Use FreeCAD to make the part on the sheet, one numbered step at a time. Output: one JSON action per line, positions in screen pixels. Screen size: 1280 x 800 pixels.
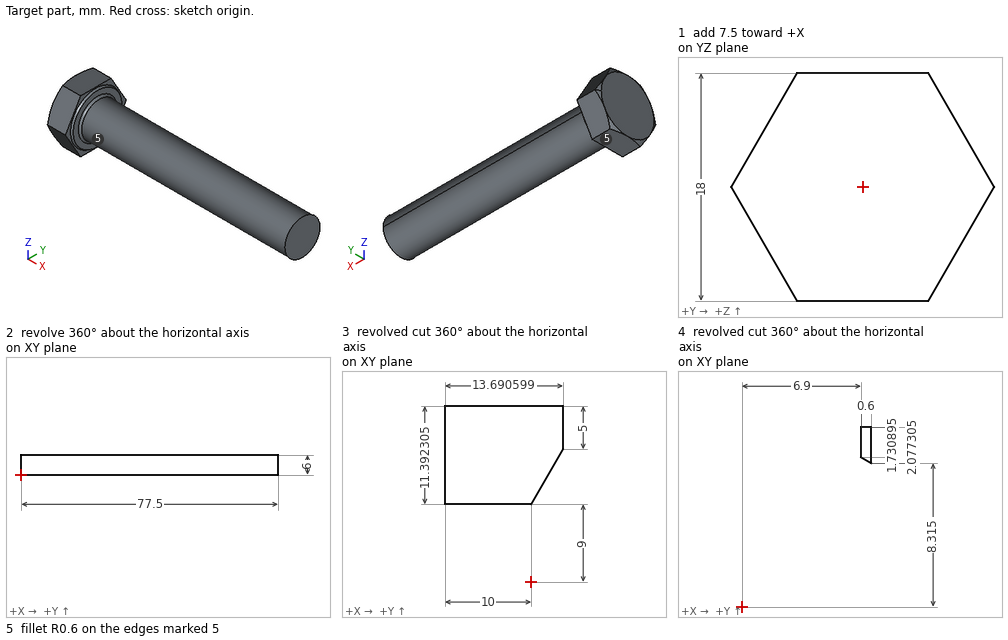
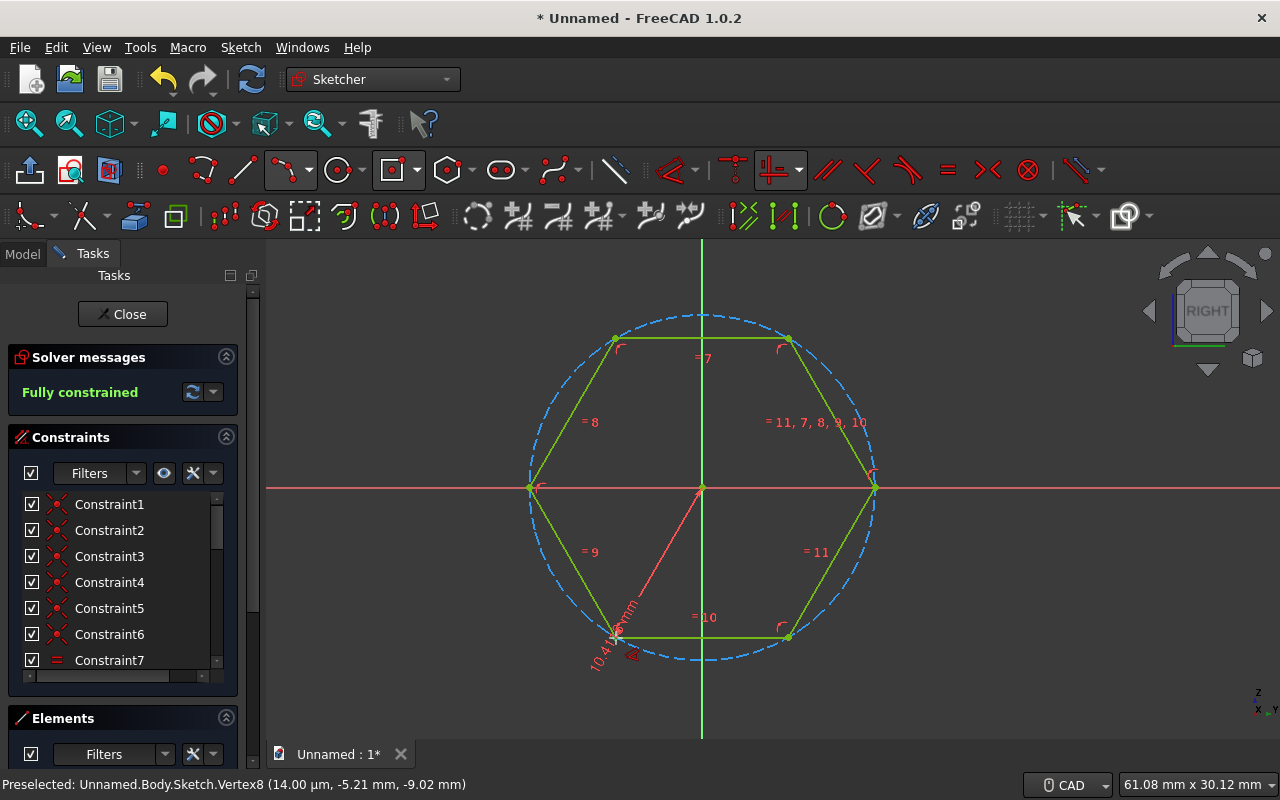
{"action": "left_click", "coordinate": [789, 338]}
{"action": "left_click", "coordinate": [871, 383]}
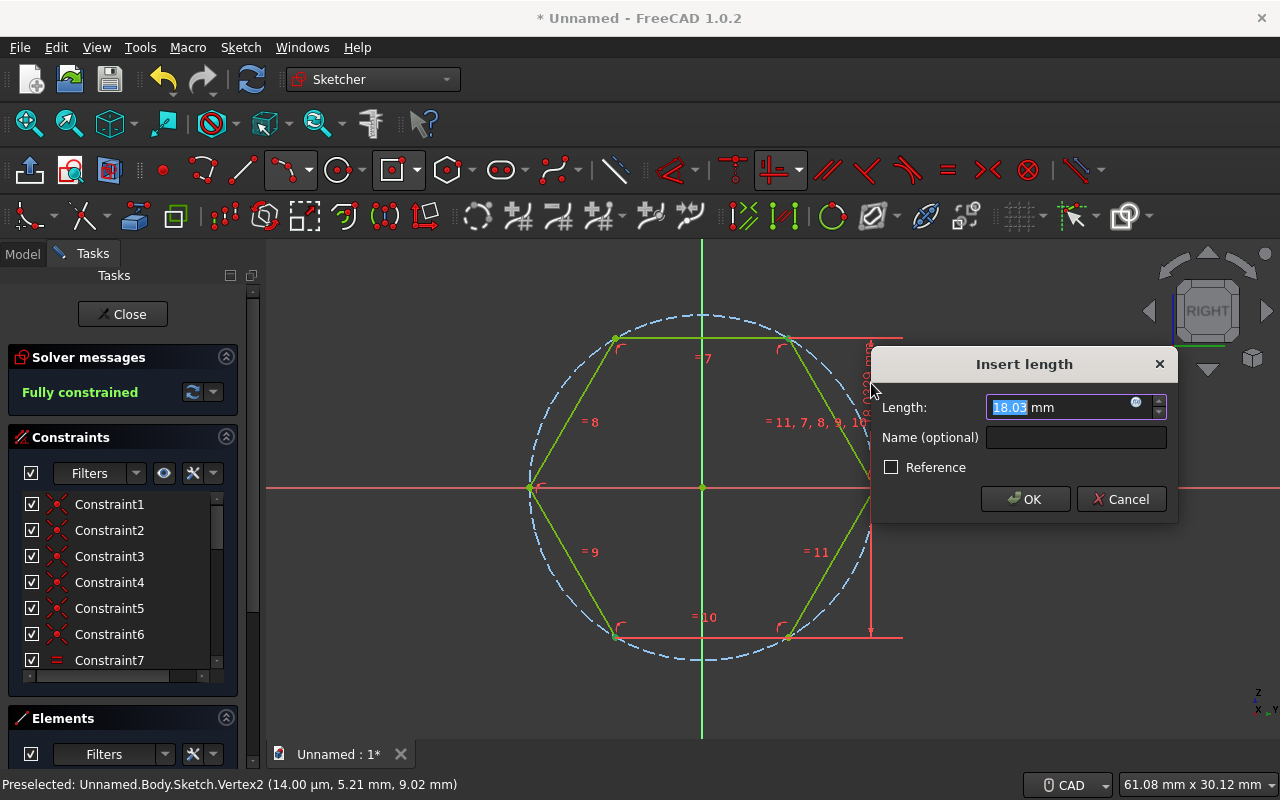
{"action": "type", "text": "18"}
{"action": "key", "text": "Return"}
{"action": "key", "text": "Escape"}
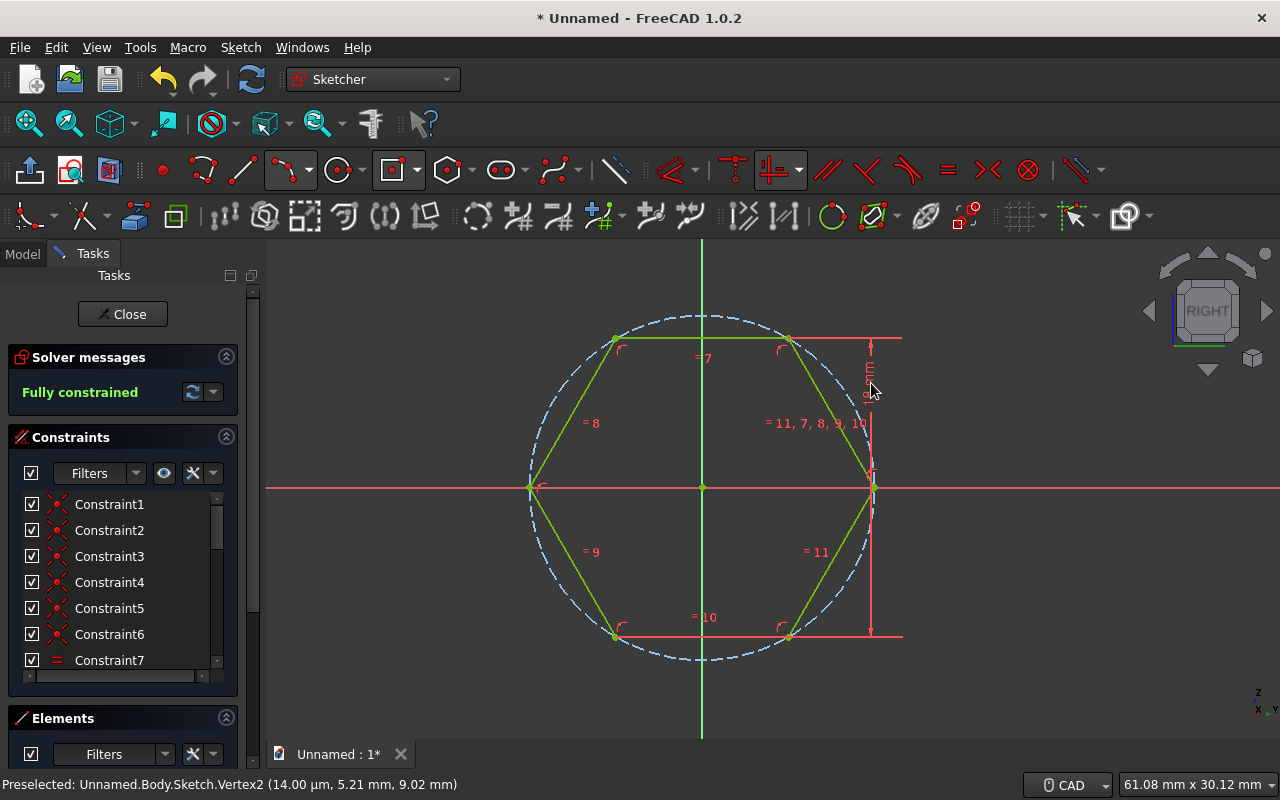
{"action": "left_click", "coordinate": [123, 314]}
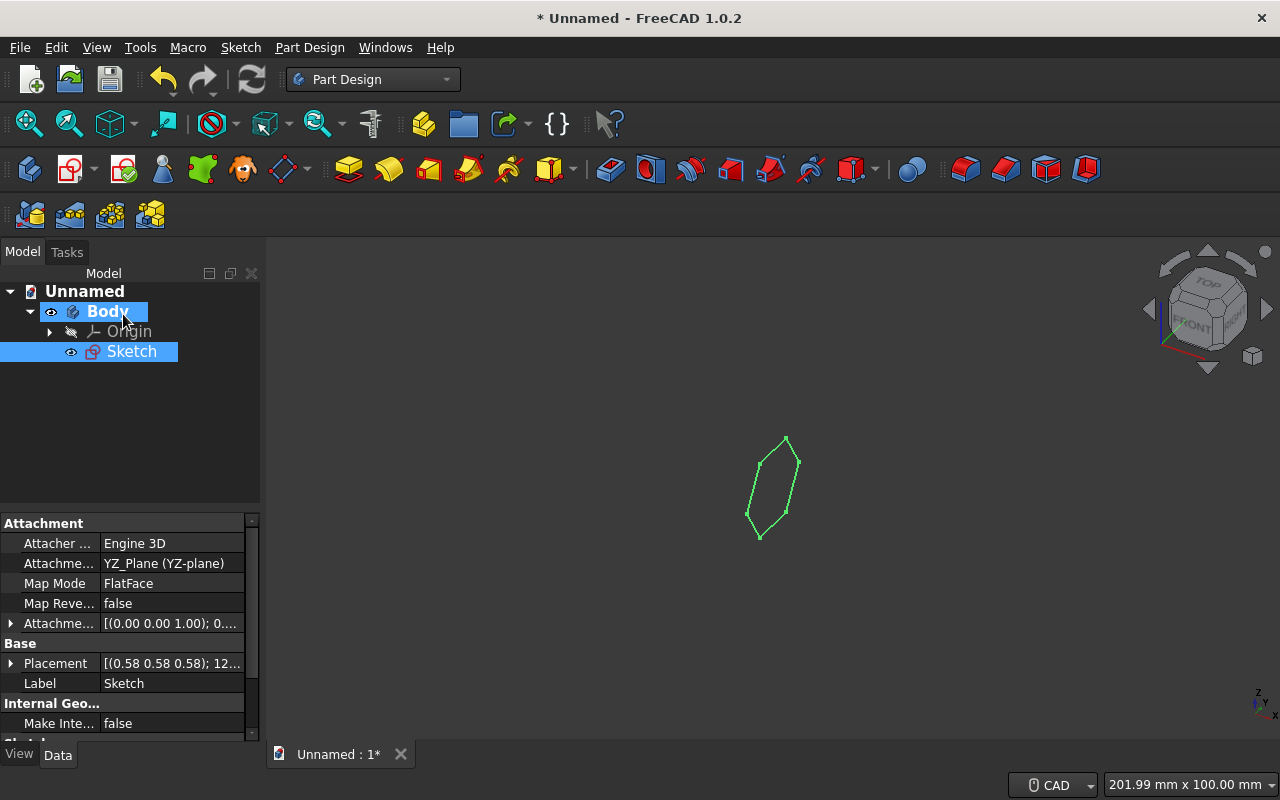
{"action": "left_click", "coordinate": [350, 170]}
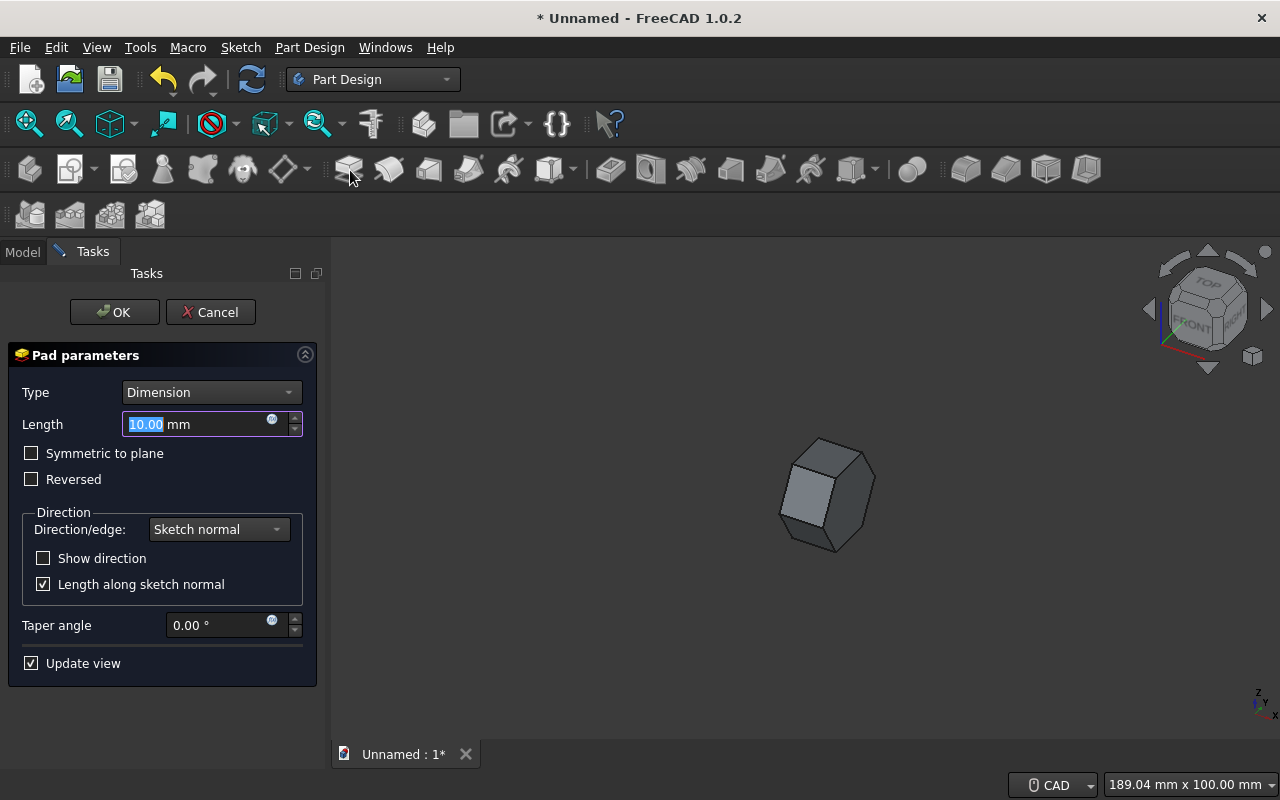
{"action": "type", "text": "7.5"}
{"action": "key", "text": "Tab"}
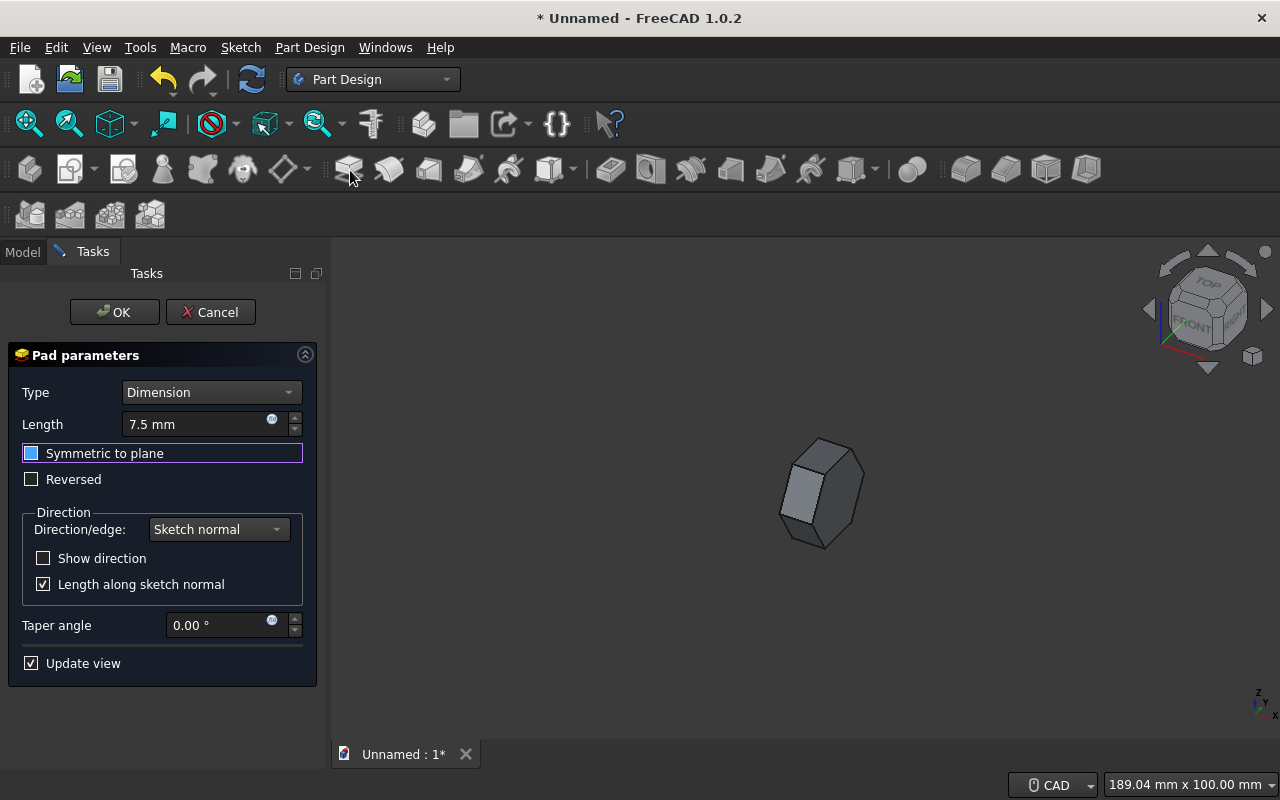
{"action": "left_click", "coordinate": [115, 312]}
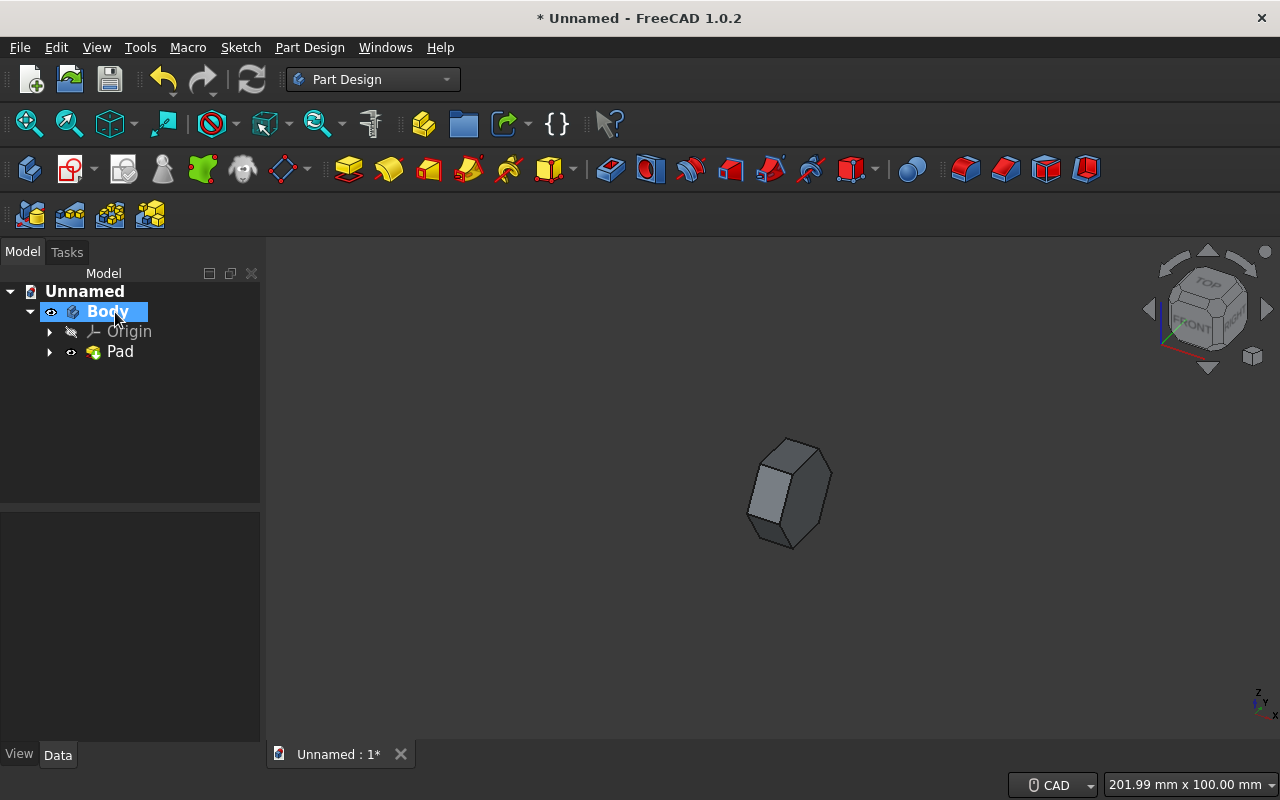
{"action": "left_click", "coordinate": [30, 124]}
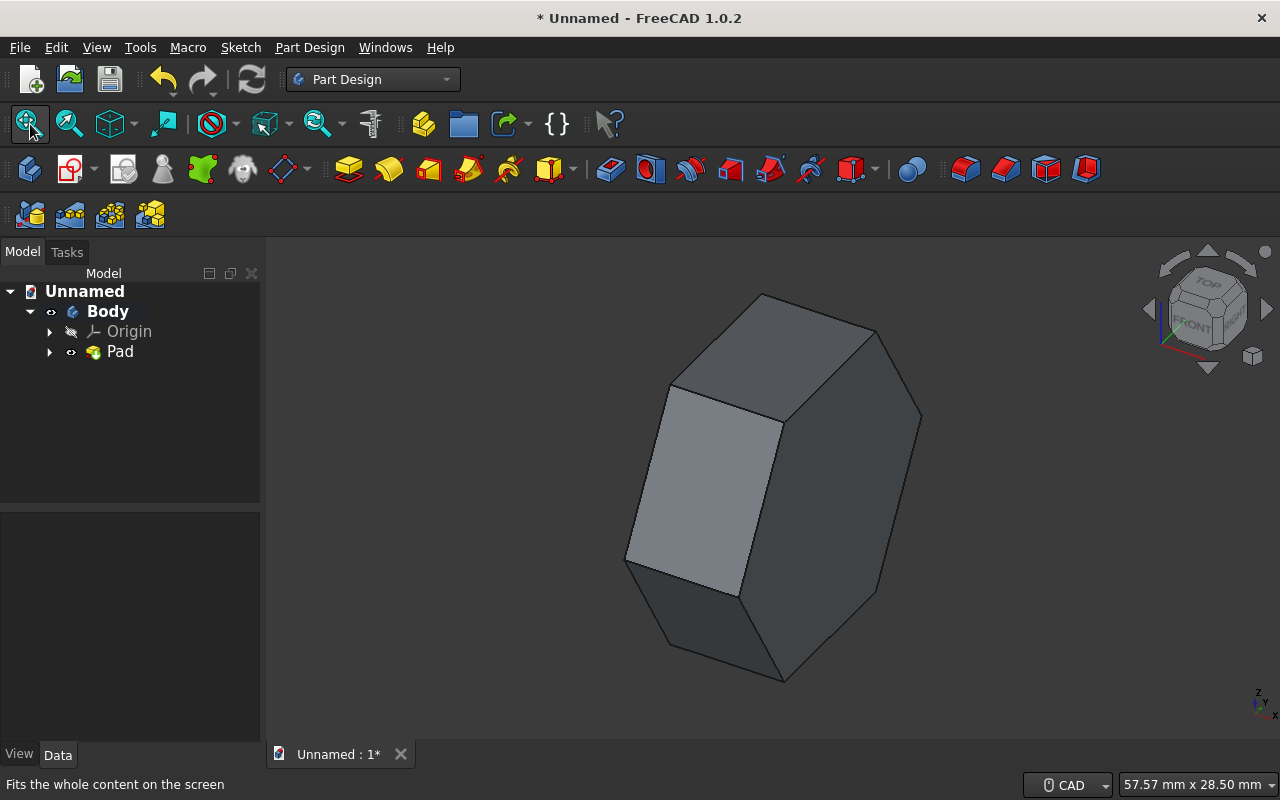
{"action": "left_click", "coordinate": [70, 170]}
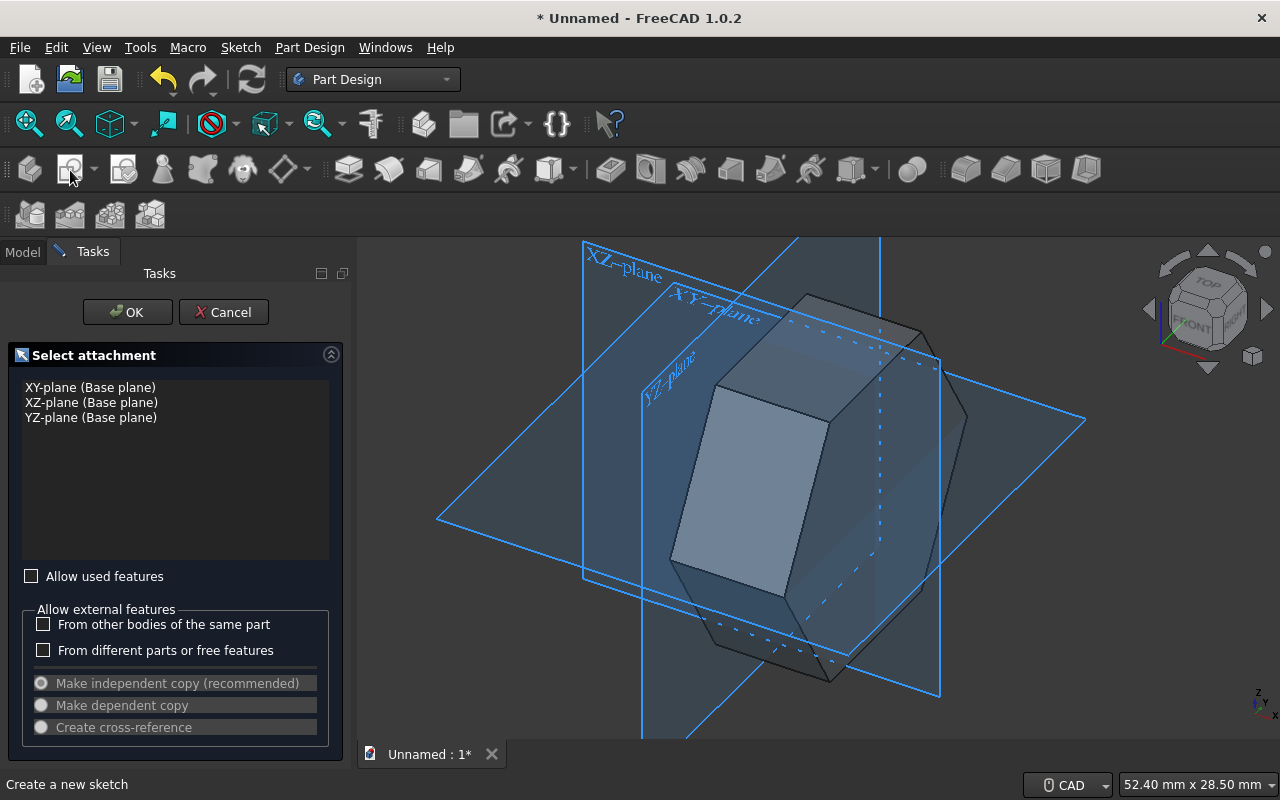
{"action": "left_click", "coordinate": [82, 388]}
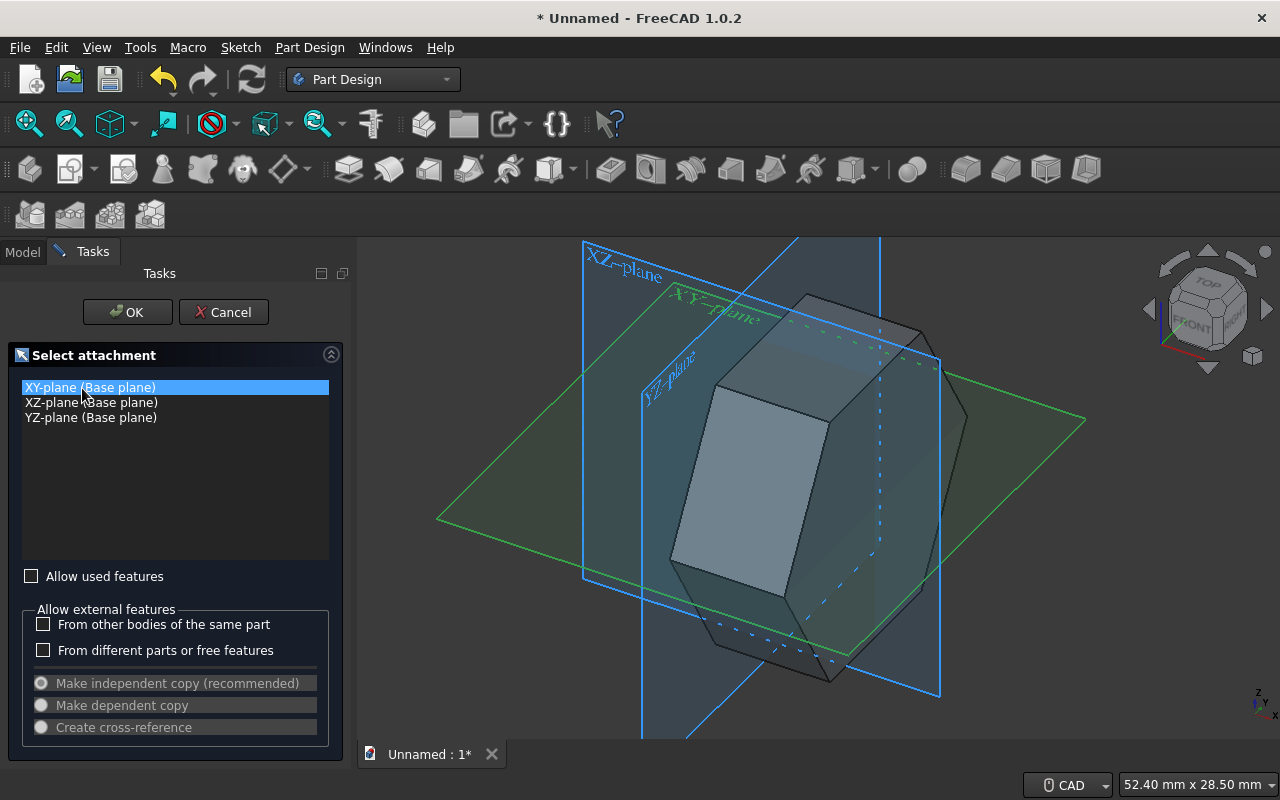
{"action": "left_click", "coordinate": [128, 312]}